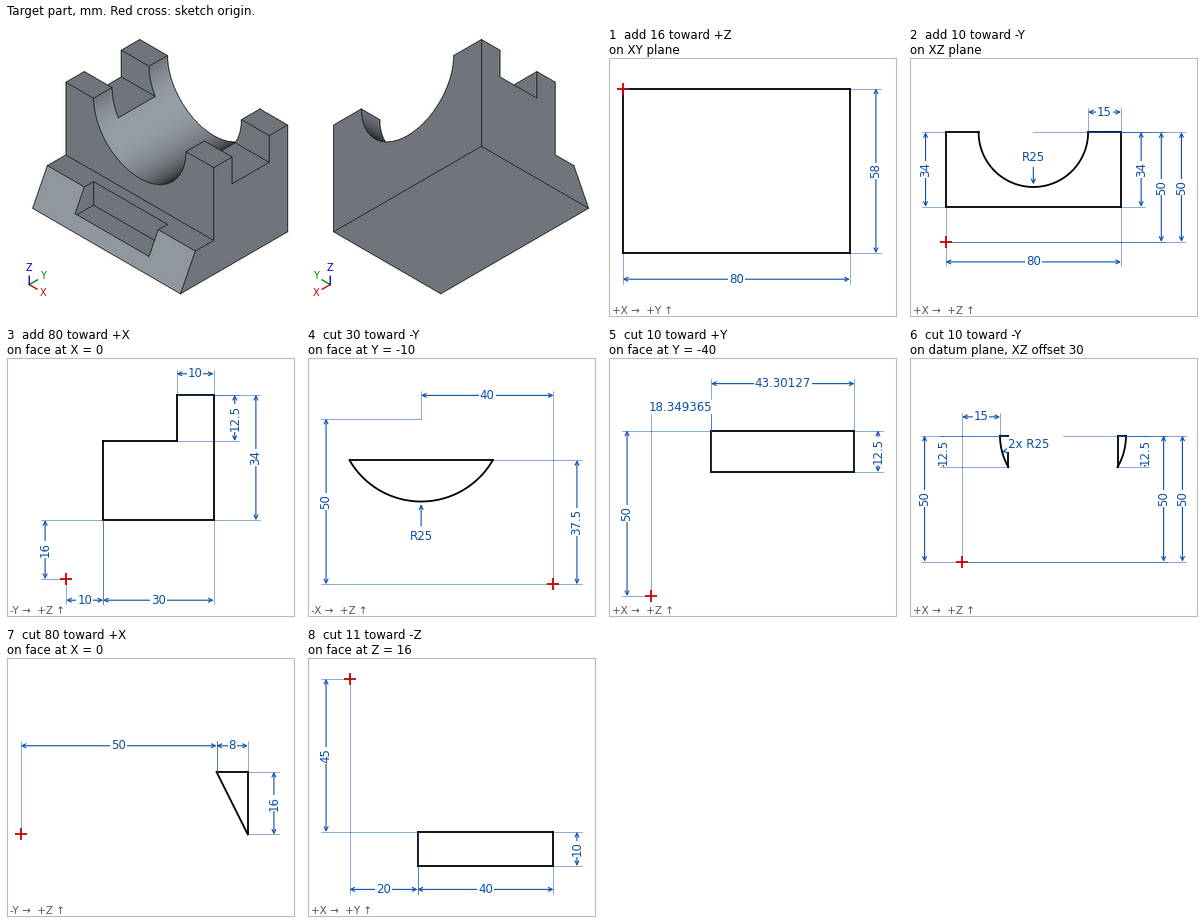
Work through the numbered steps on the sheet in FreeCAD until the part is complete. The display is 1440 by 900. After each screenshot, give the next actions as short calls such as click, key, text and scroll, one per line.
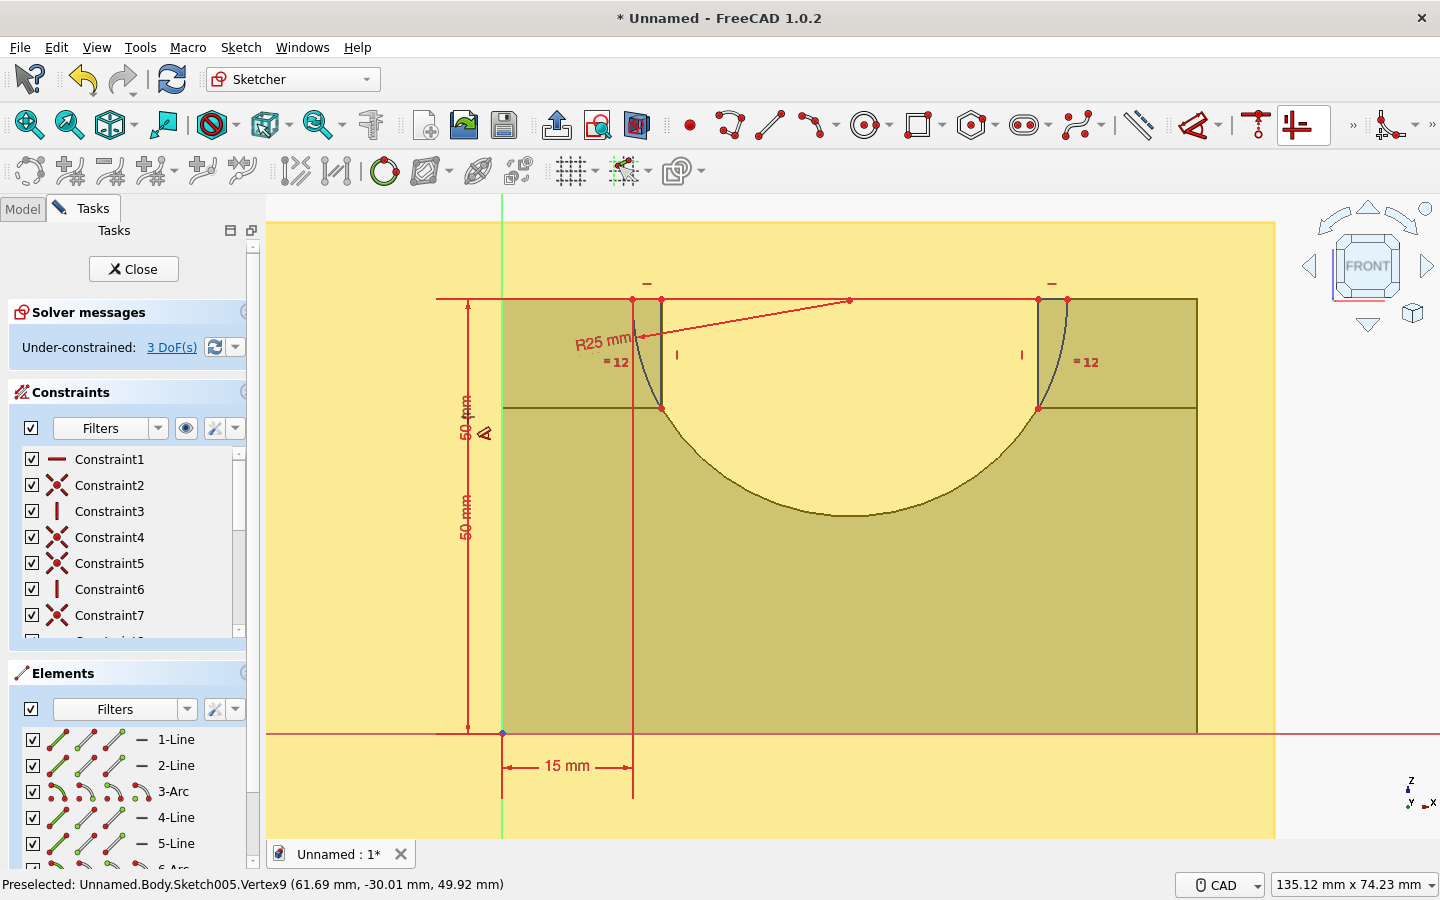
click(850, 301)
click(468, 617)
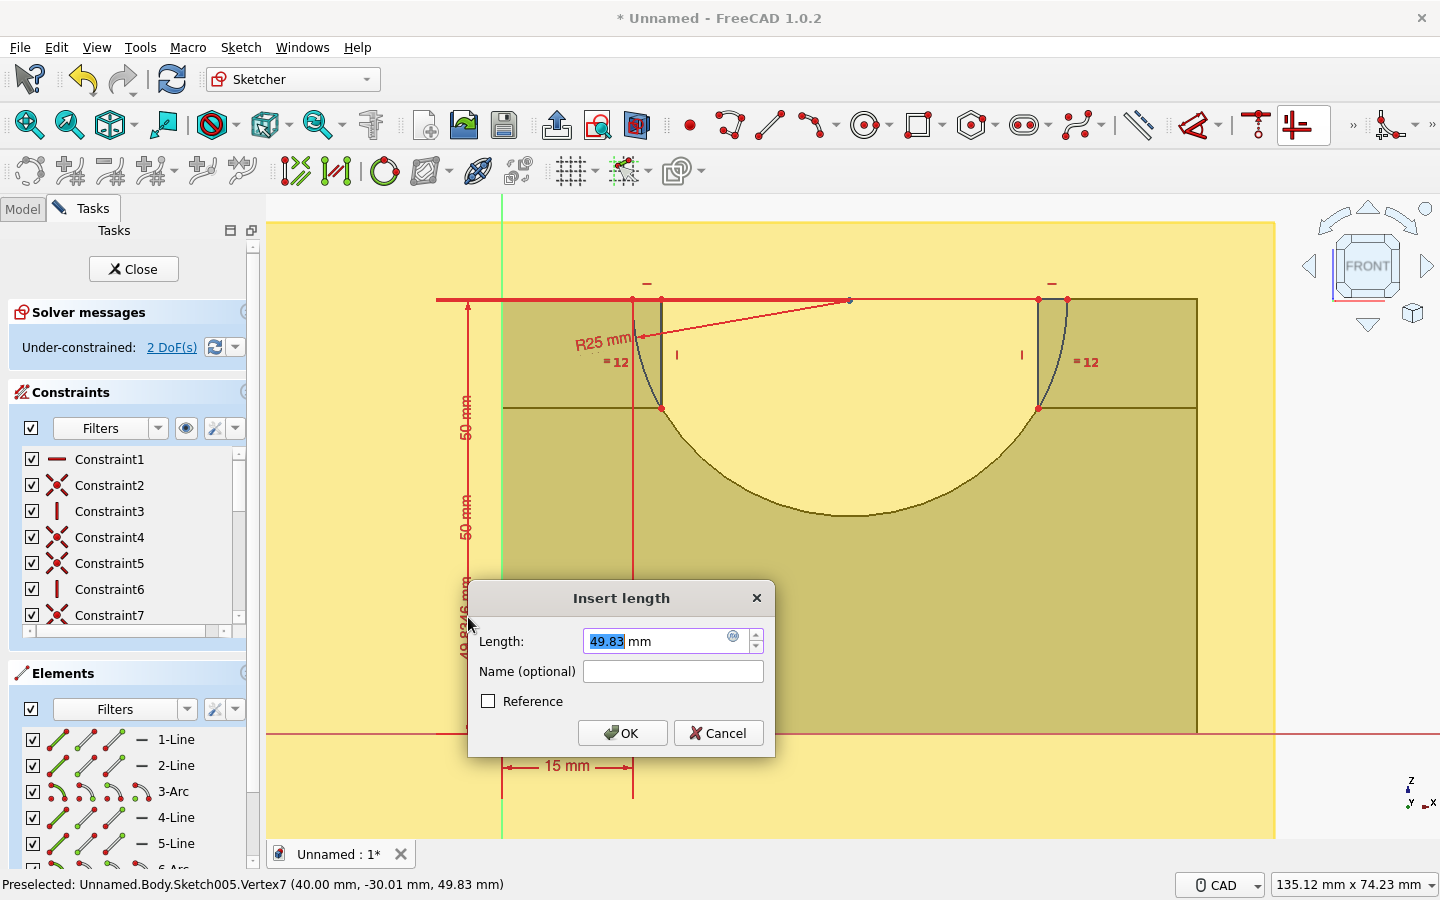
text(50)
key(Return)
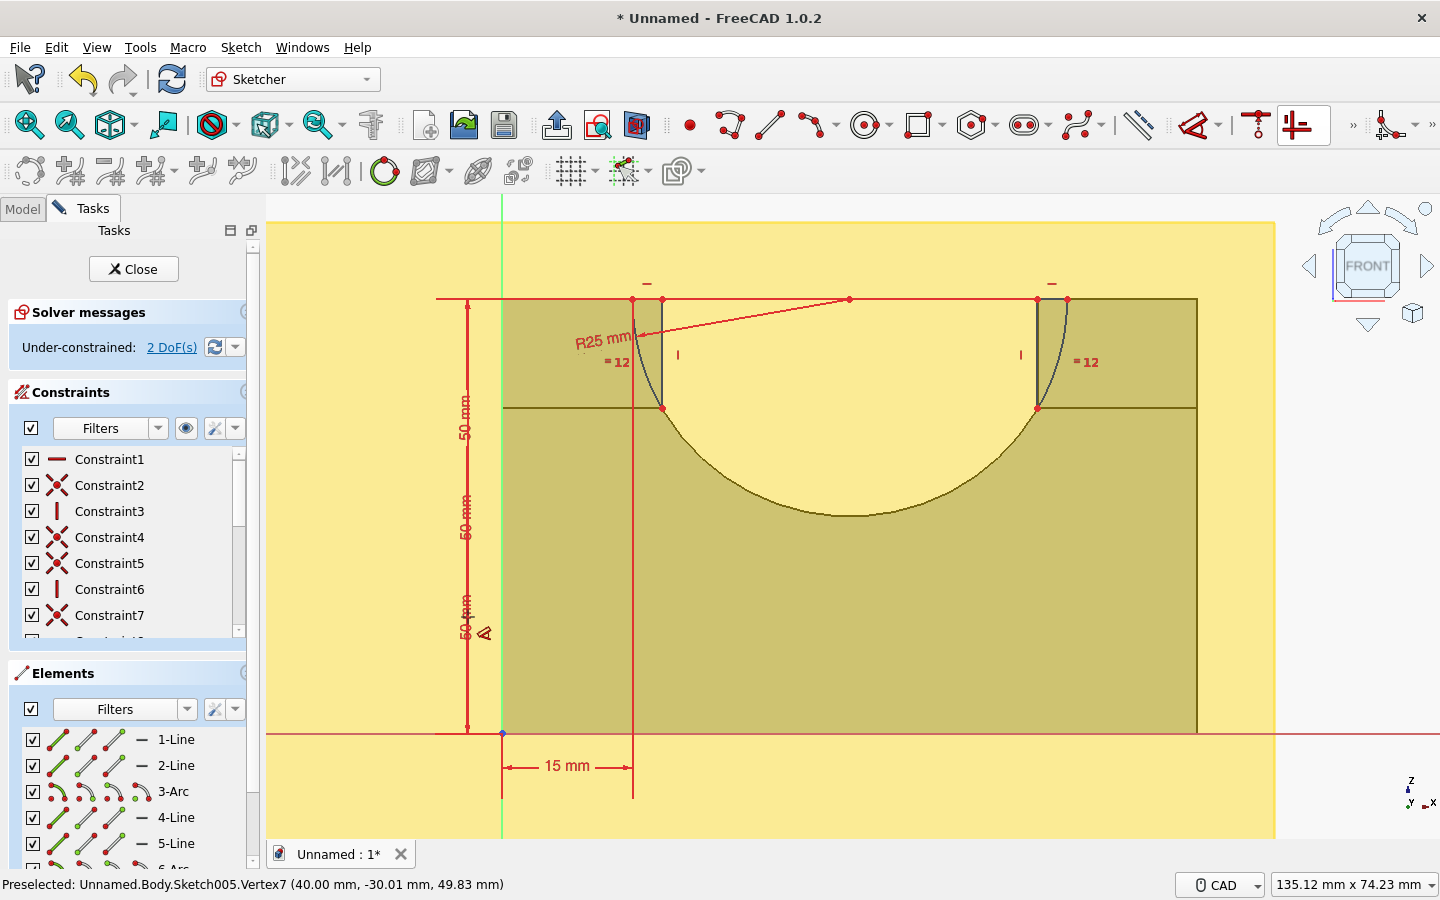
click(662, 332)
click(628, 379)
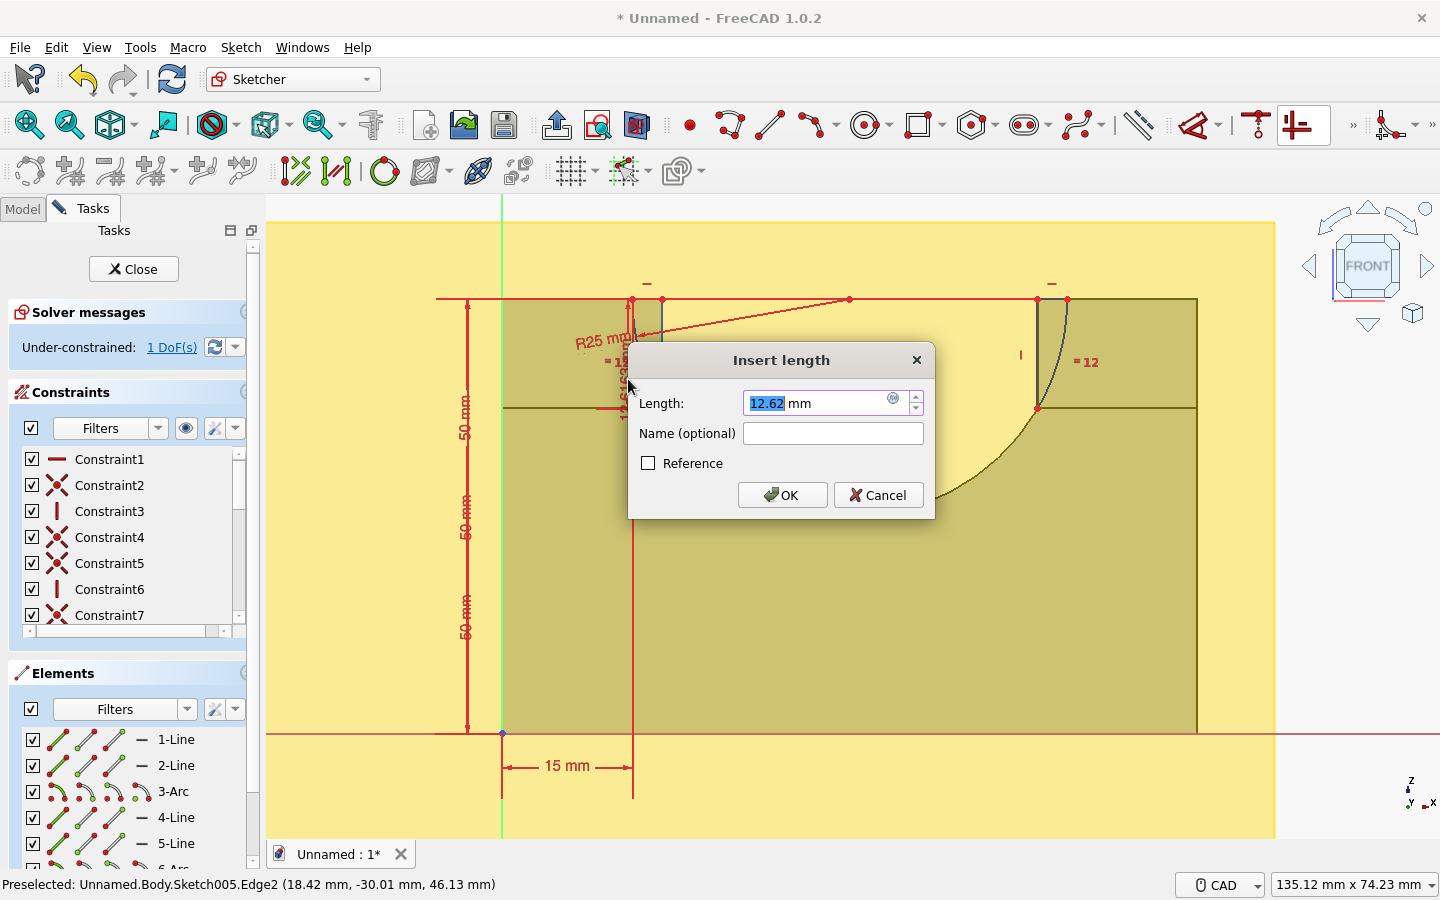
text(12.5)
key(Return)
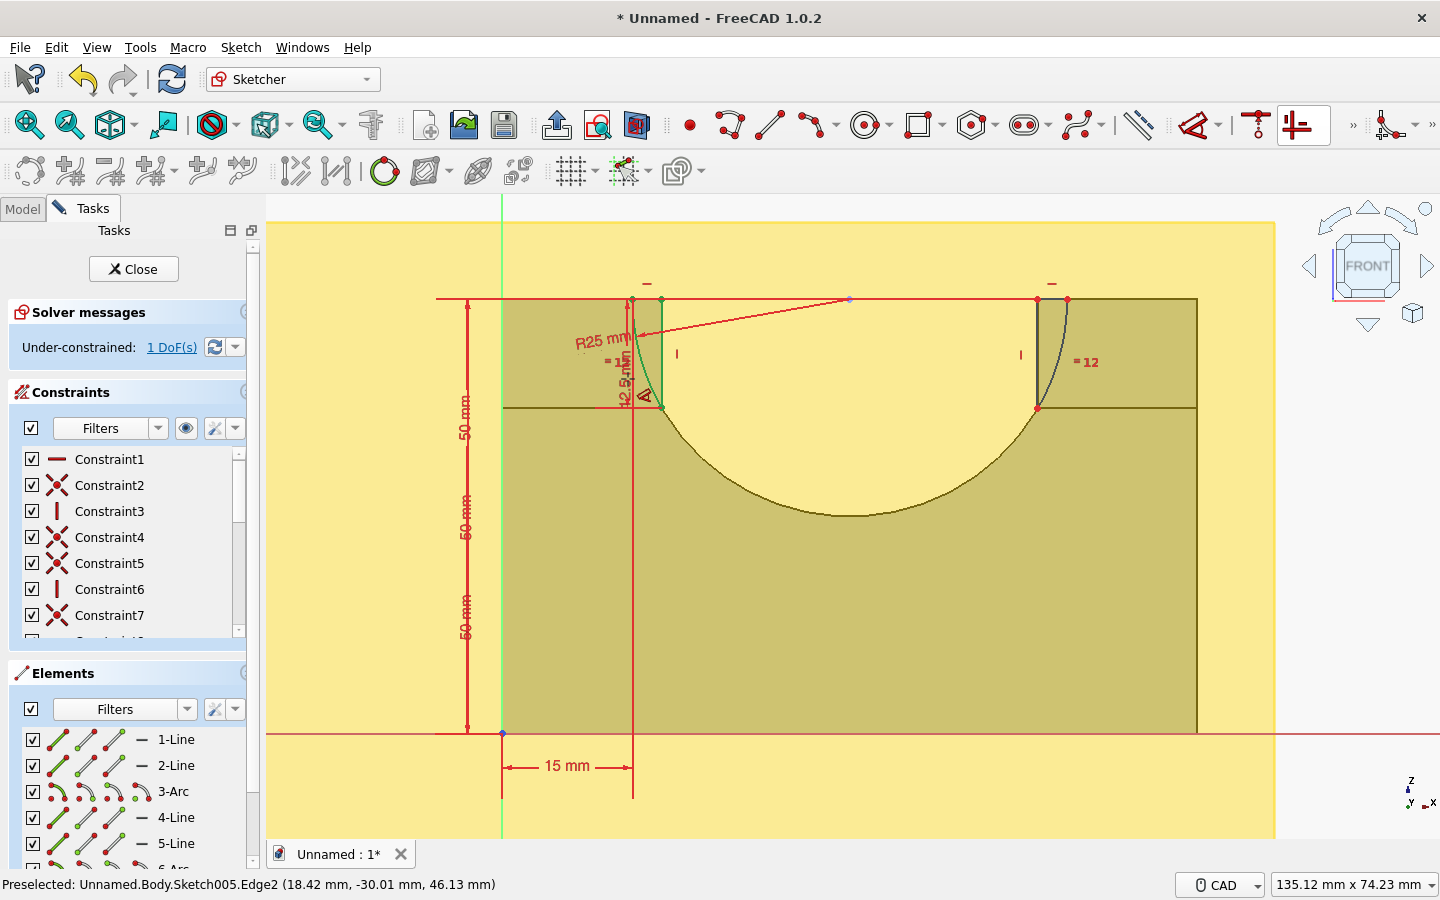
click(1037, 376)
click(1071, 379)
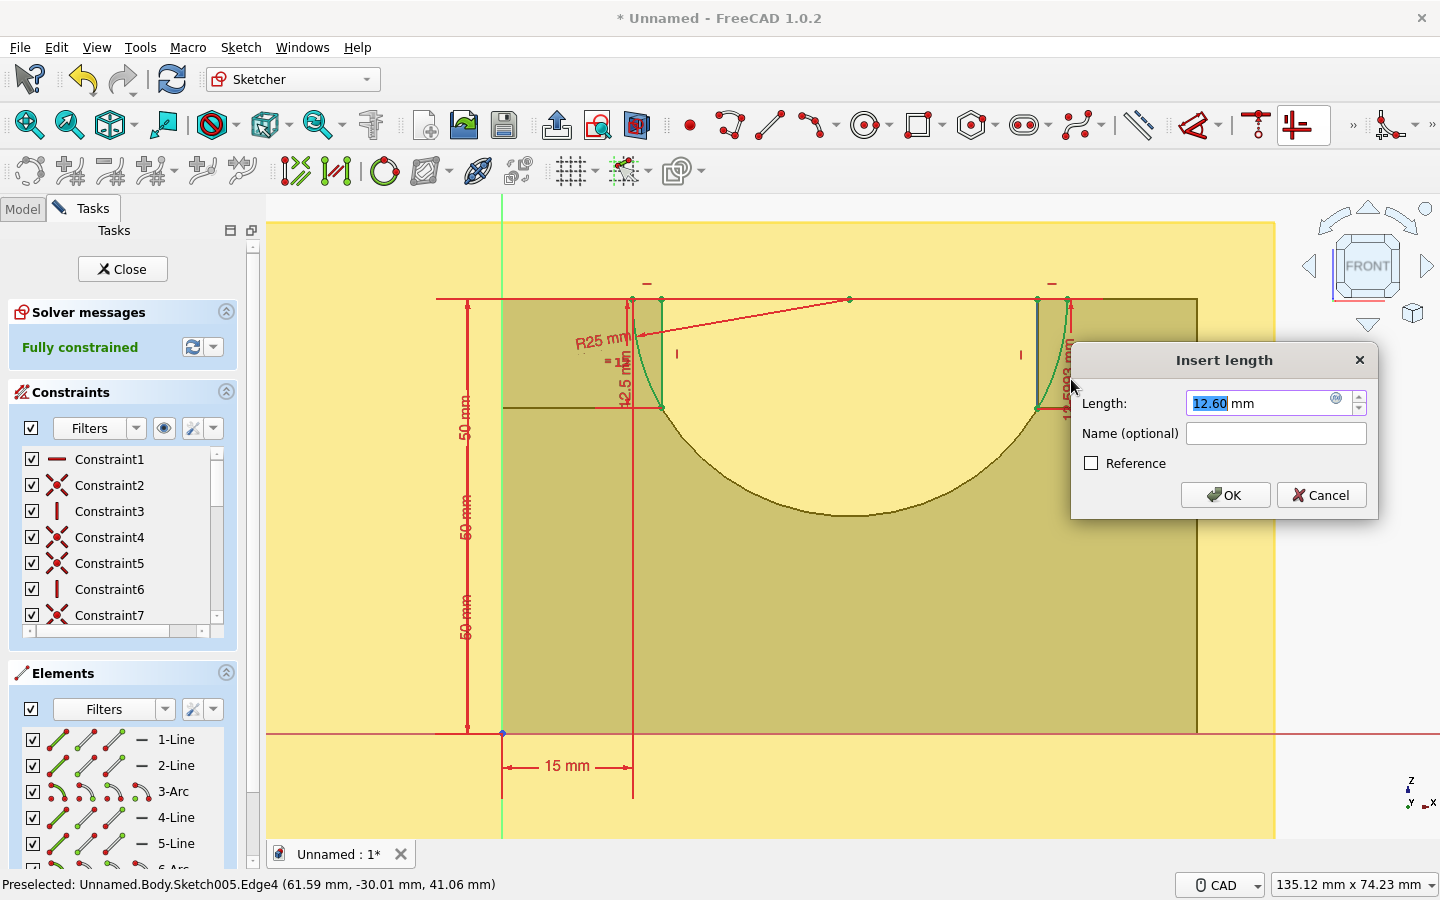
text(12.5)
key(Return)
key(Escape)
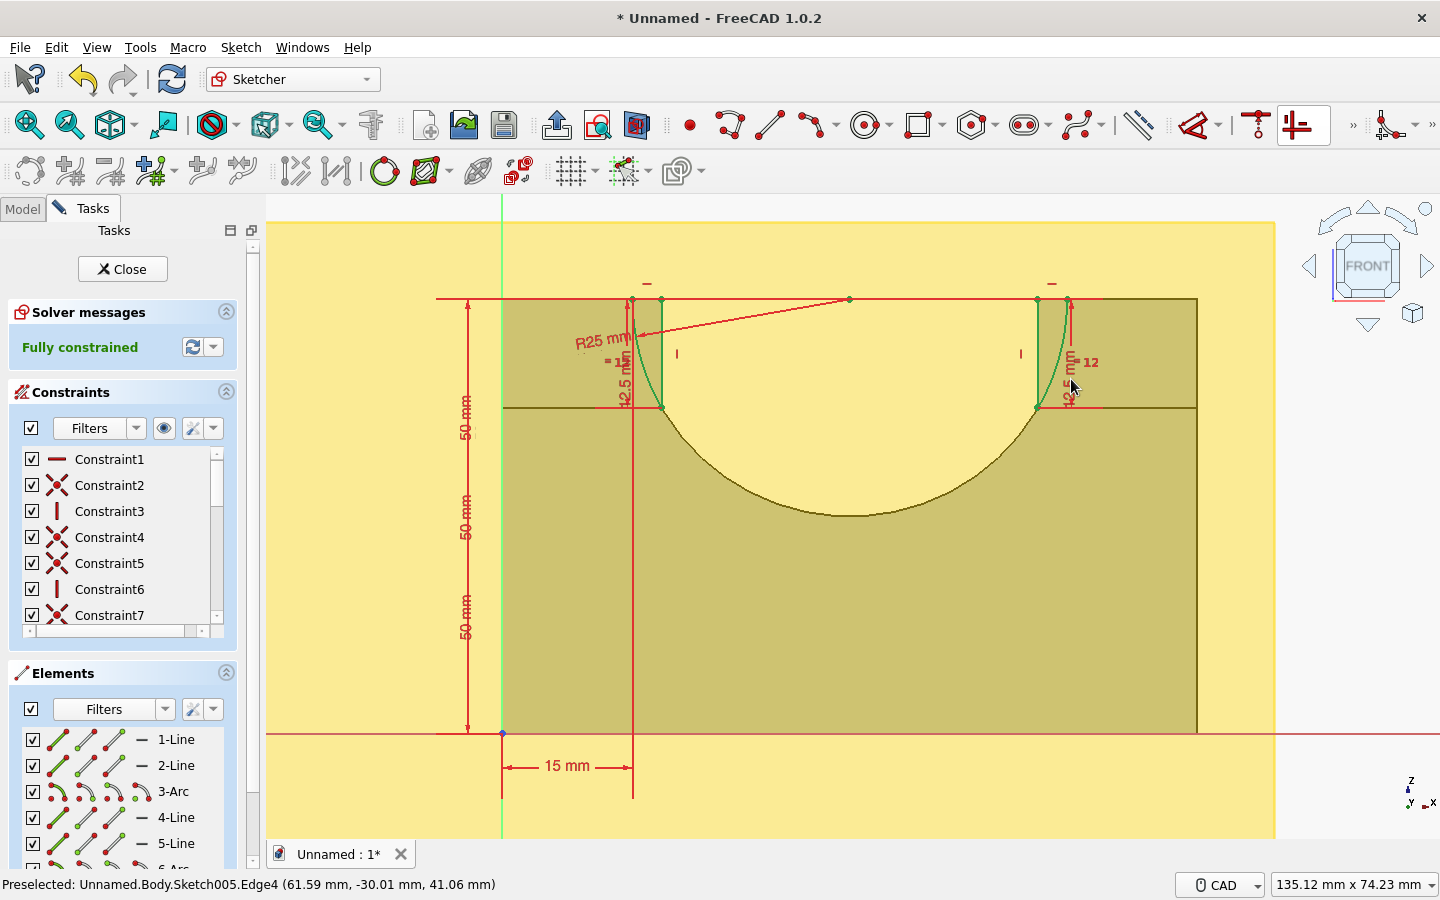
click(123, 269)